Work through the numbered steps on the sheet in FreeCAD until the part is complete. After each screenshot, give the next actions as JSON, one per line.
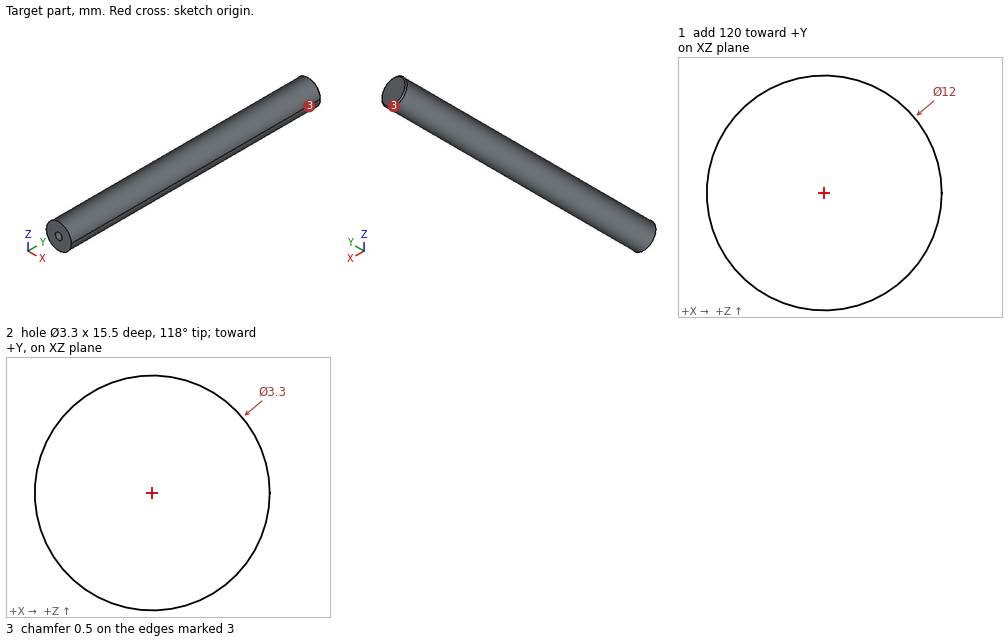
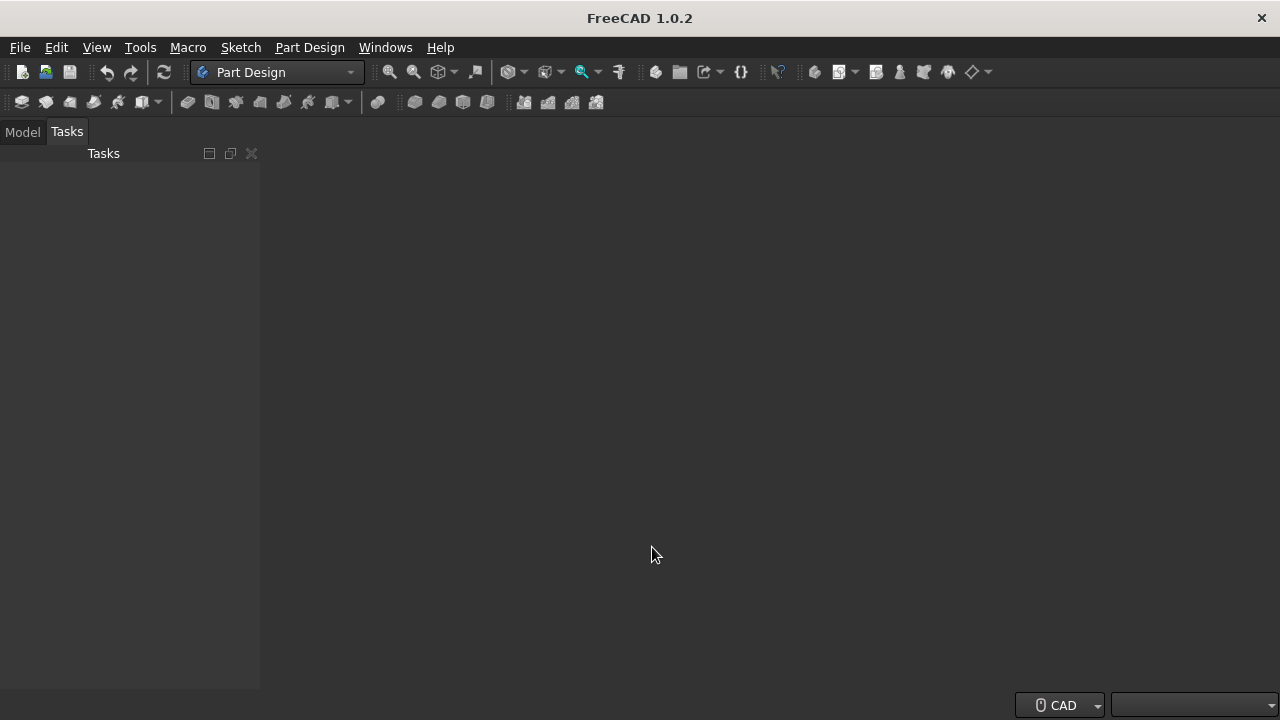
{"action": "left_click", "coordinate": [22, 72]}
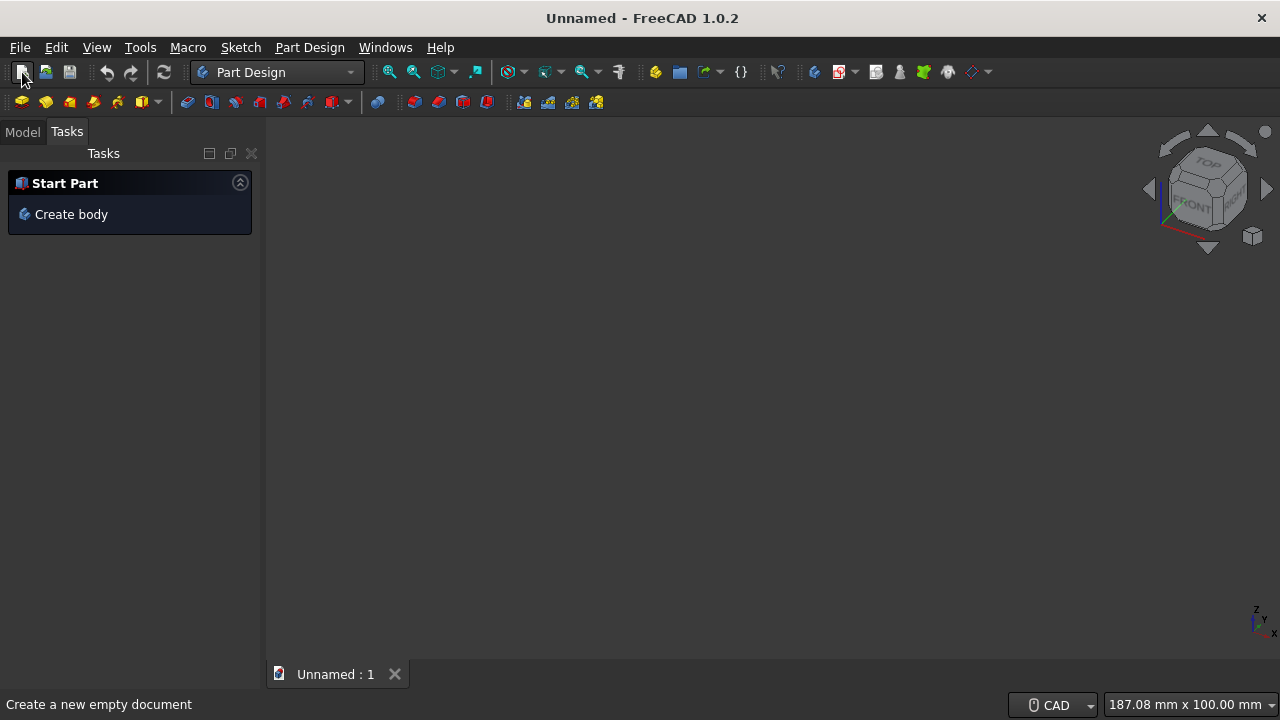
{"action": "left_click", "coordinate": [840, 72]}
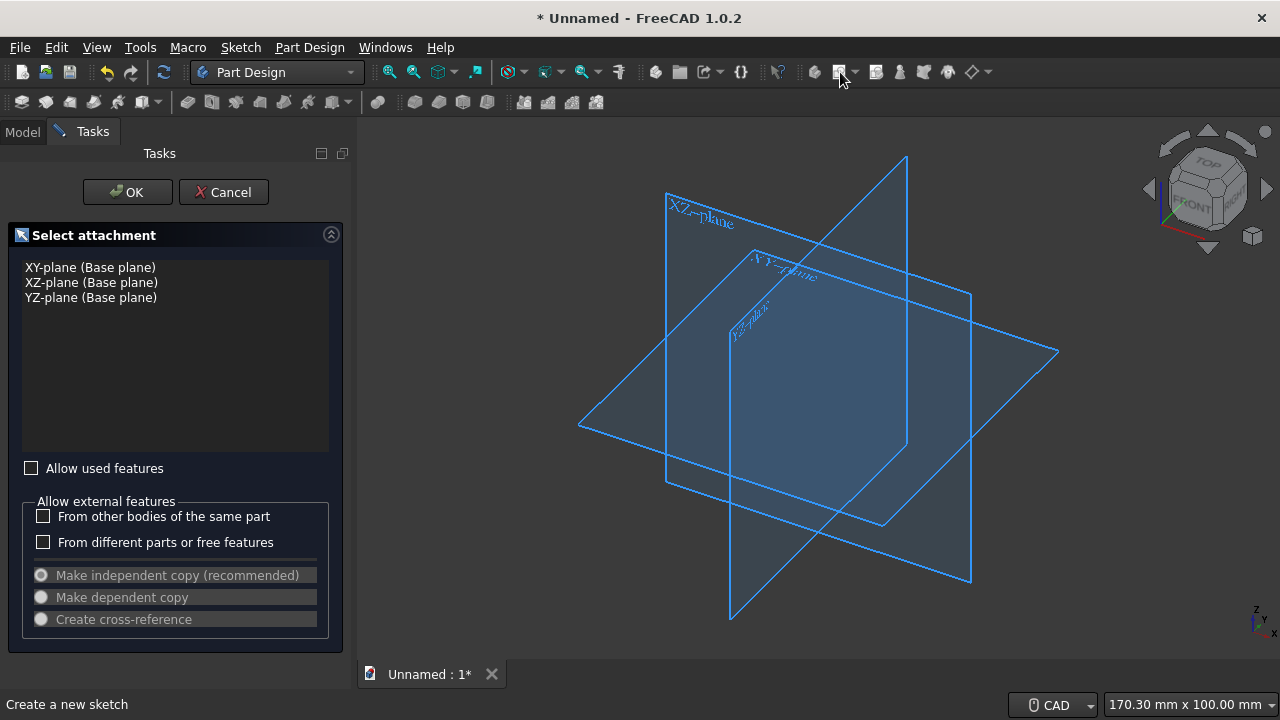
{"action": "left_click", "coordinate": [82, 282]}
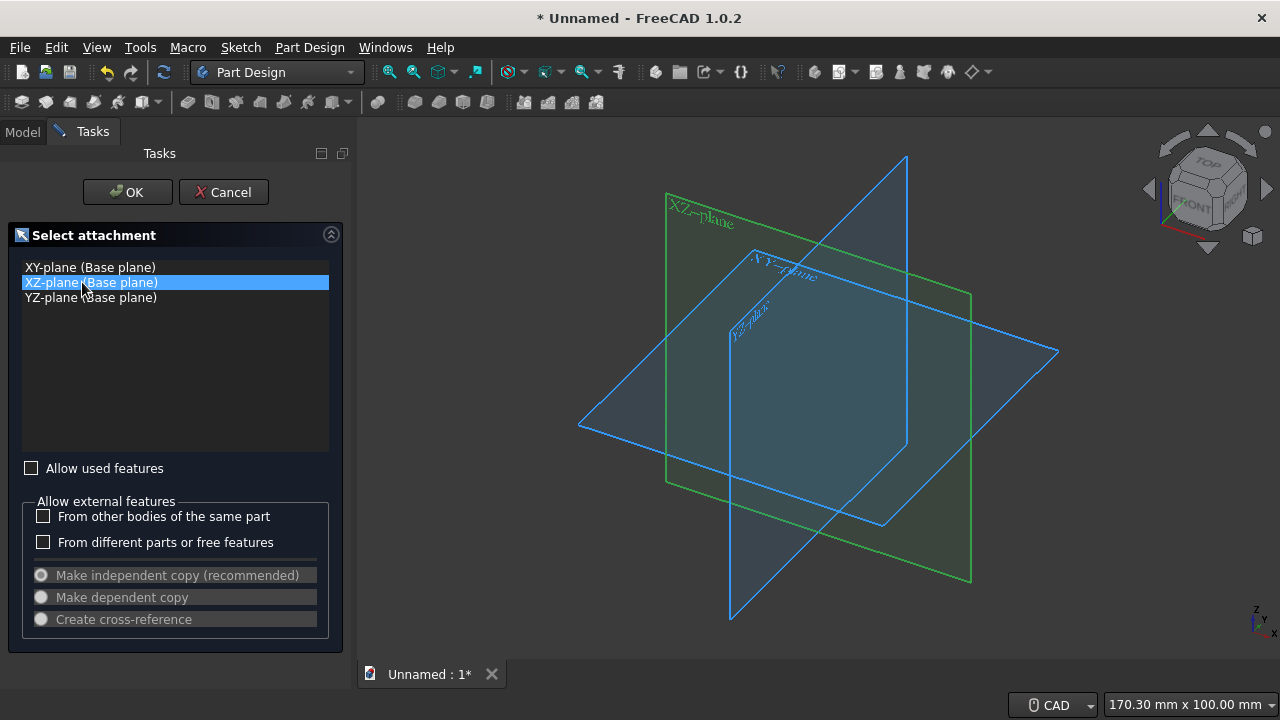
{"action": "left_click", "coordinate": [128, 192]}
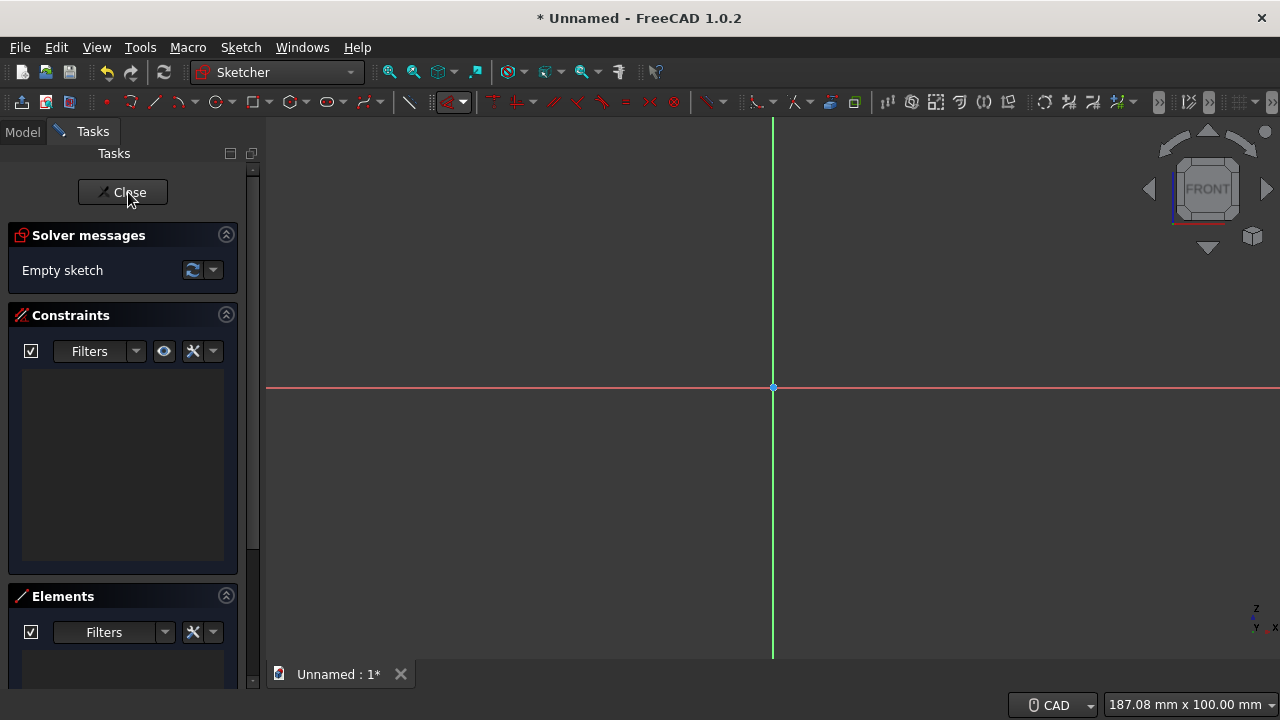
{"action": "scroll", "coordinate": [790, 388], "scroll_direction": "up", "scroll_amount": 8}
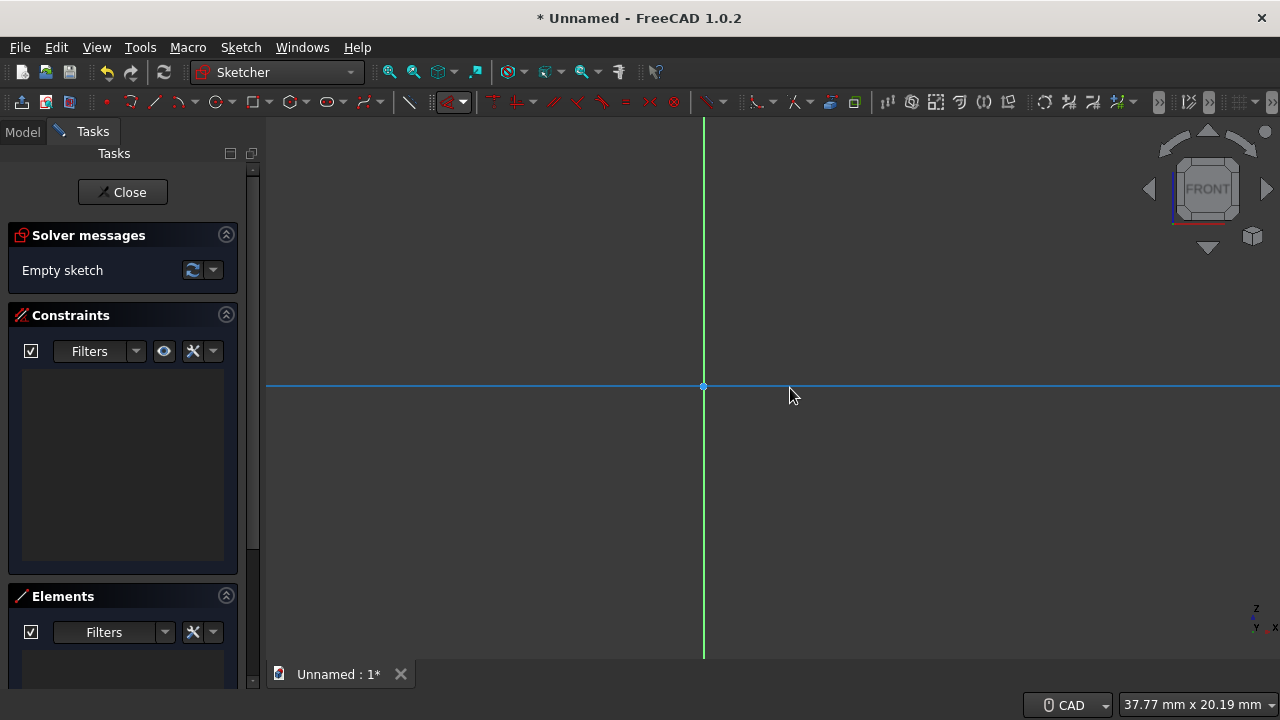
{"action": "left_click", "coordinate": [216, 102]}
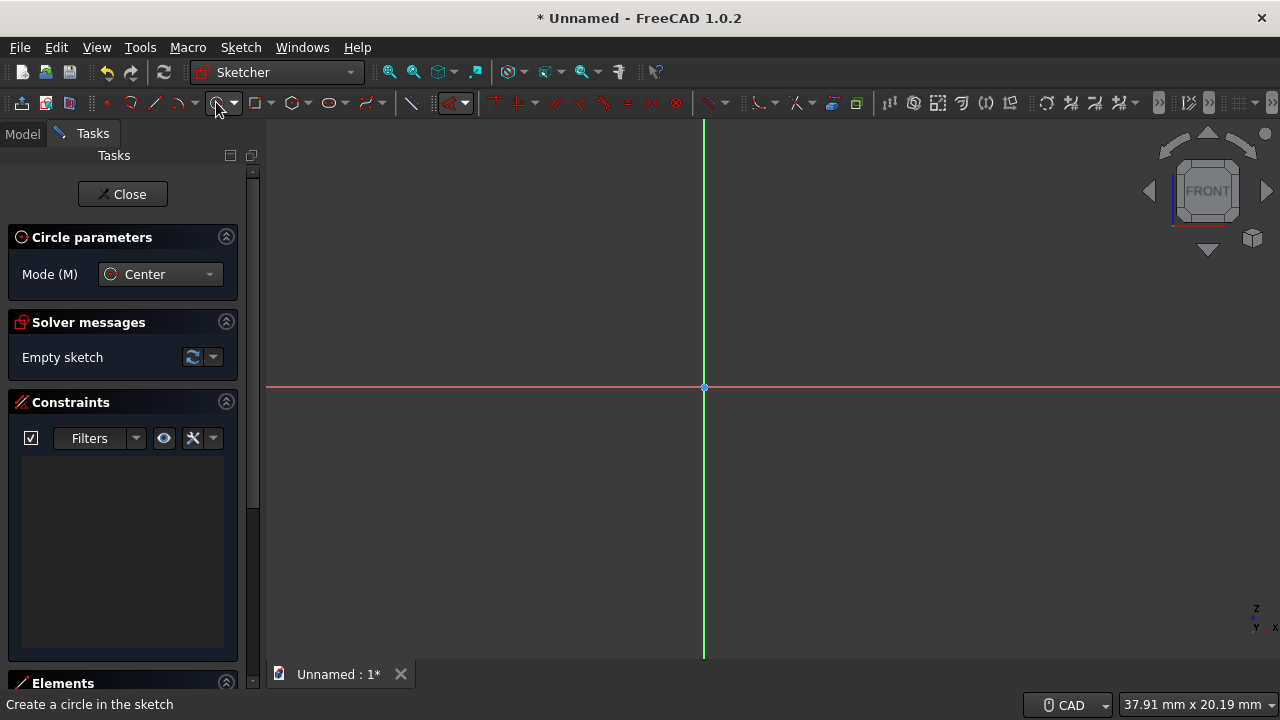
{"action": "left_click", "coordinate": [704, 387]}
{"action": "left_click", "coordinate": [817, 274]}
{"action": "key", "text": "Escape"}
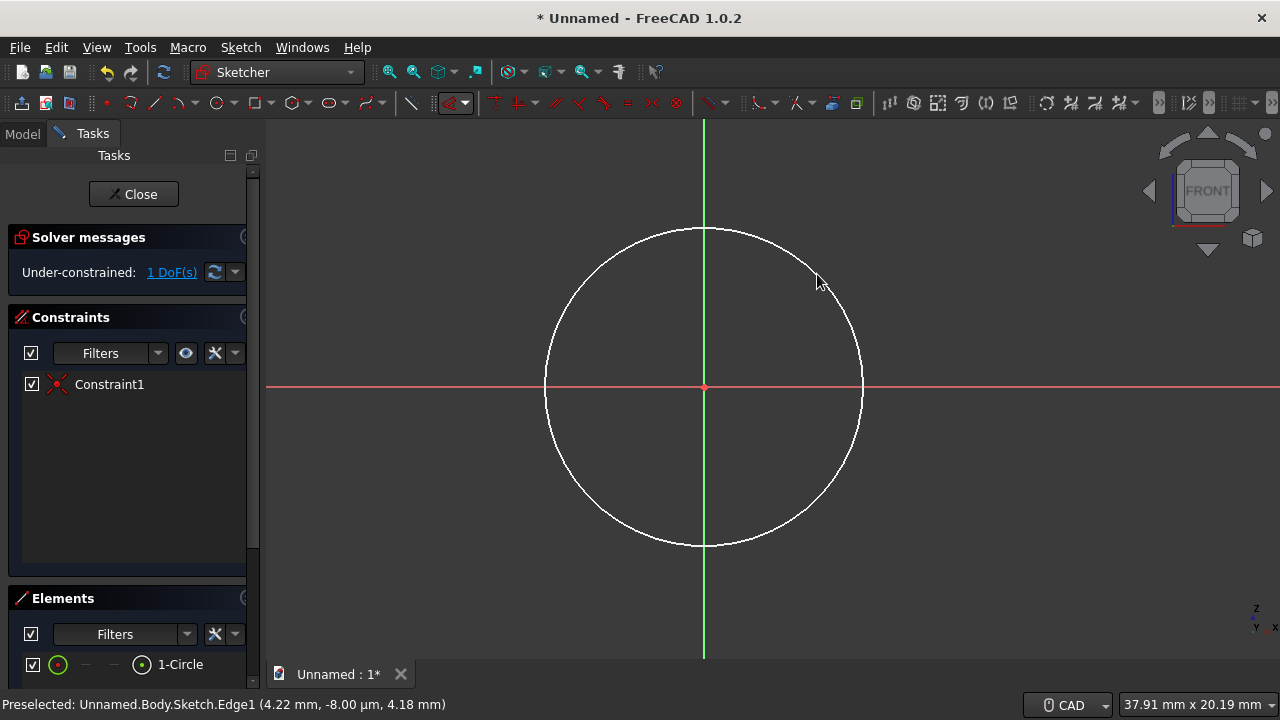
{"action": "left_click", "coordinate": [450, 104]}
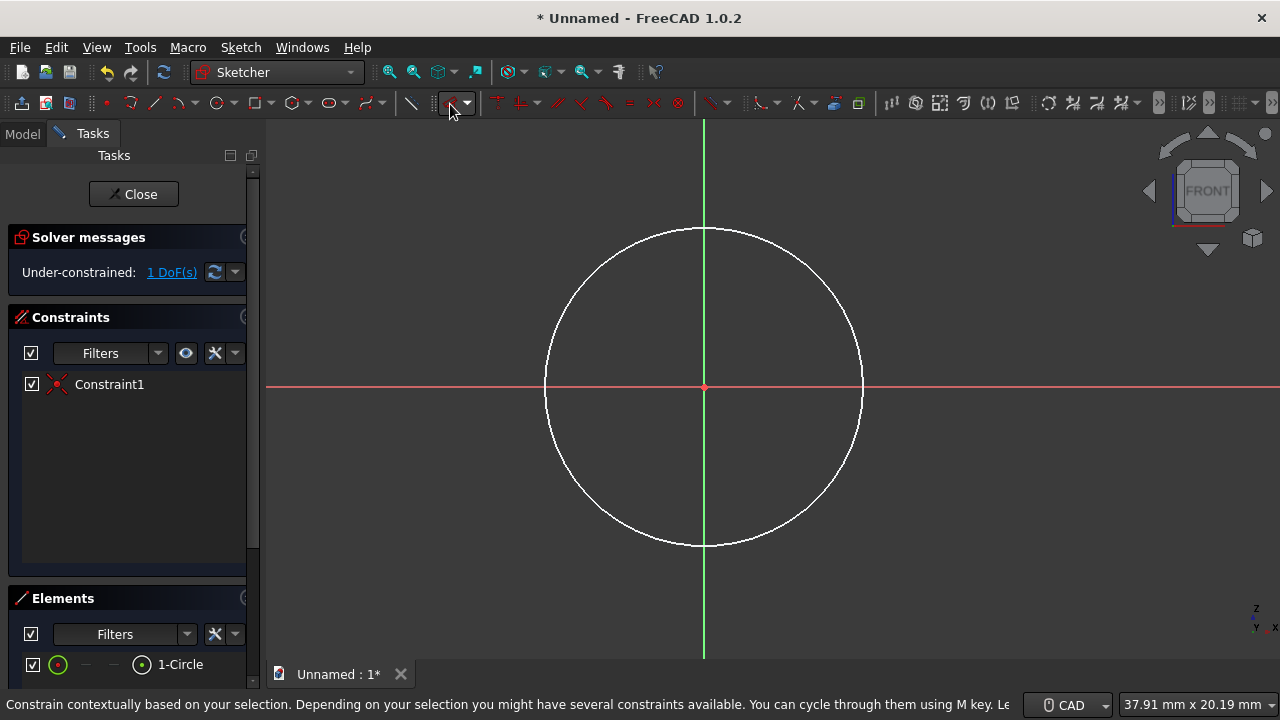
{"action": "left_click", "coordinate": [816, 274]}
{"action": "left_click", "coordinate": [839, 251]}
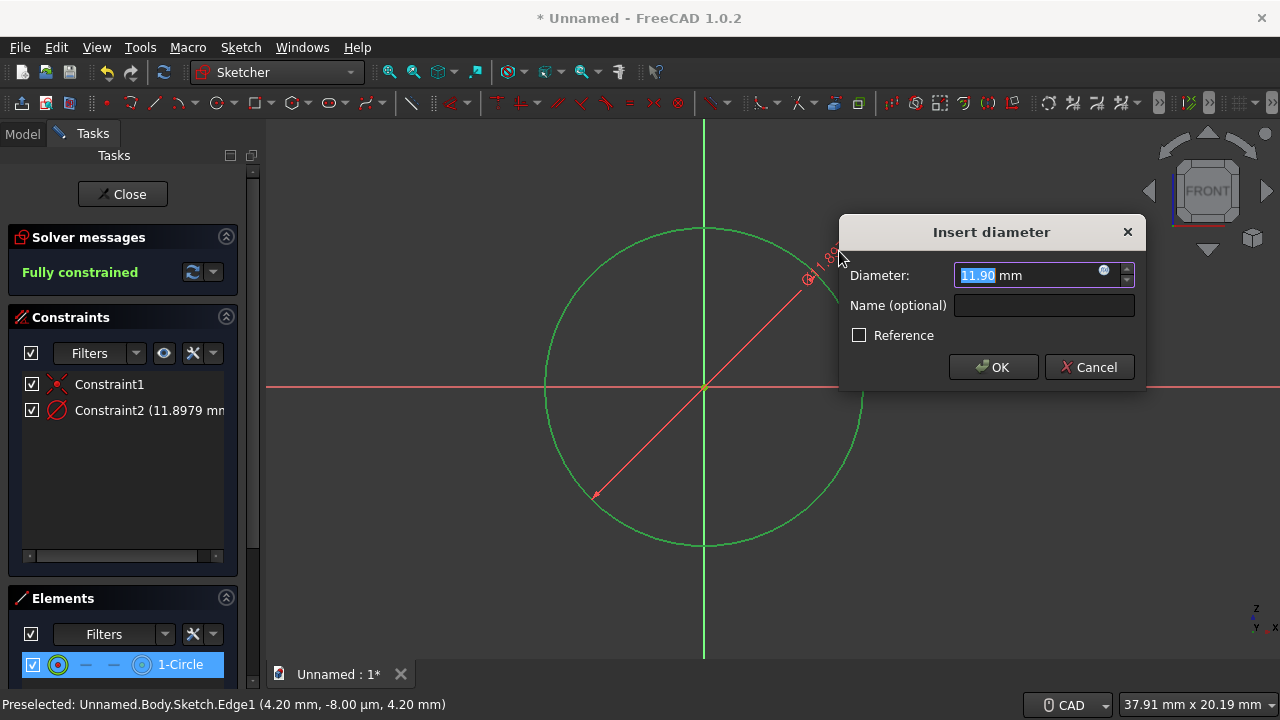
{"action": "type", "text": "12"}
{"action": "key", "text": "Return"}
{"action": "key", "text": "Escape"}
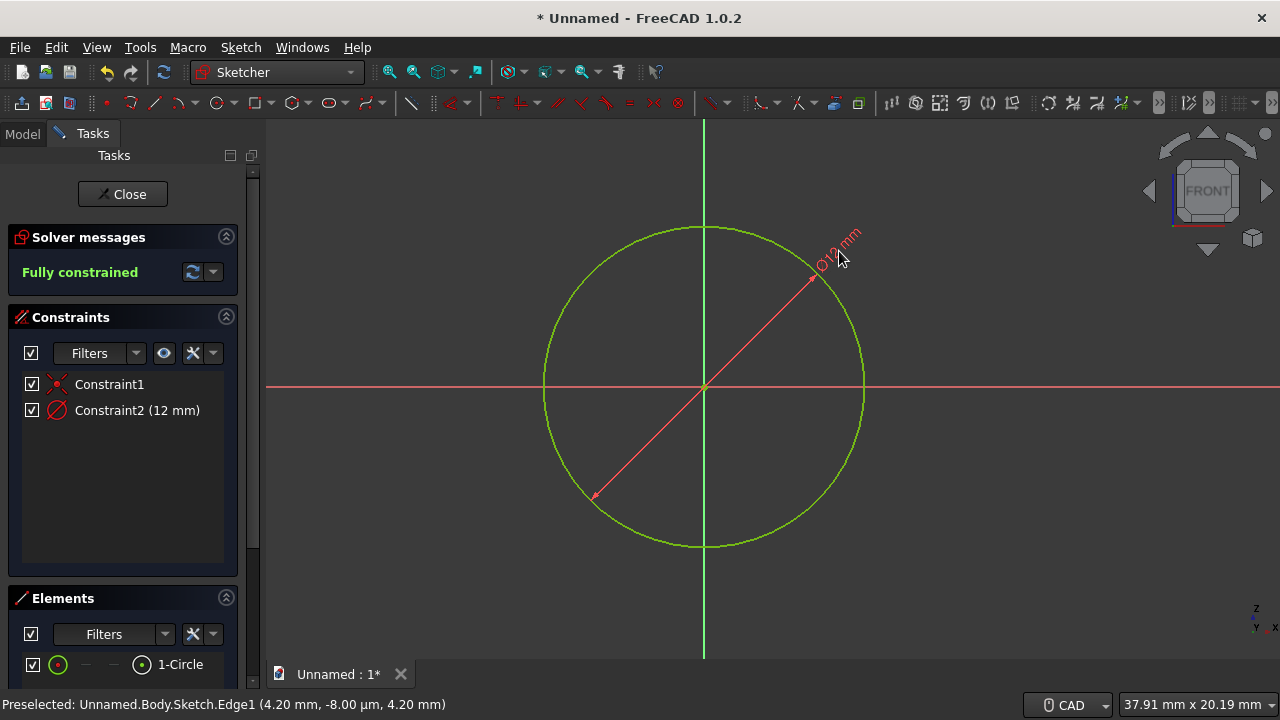
{"action": "left_click", "coordinate": [123, 194]}